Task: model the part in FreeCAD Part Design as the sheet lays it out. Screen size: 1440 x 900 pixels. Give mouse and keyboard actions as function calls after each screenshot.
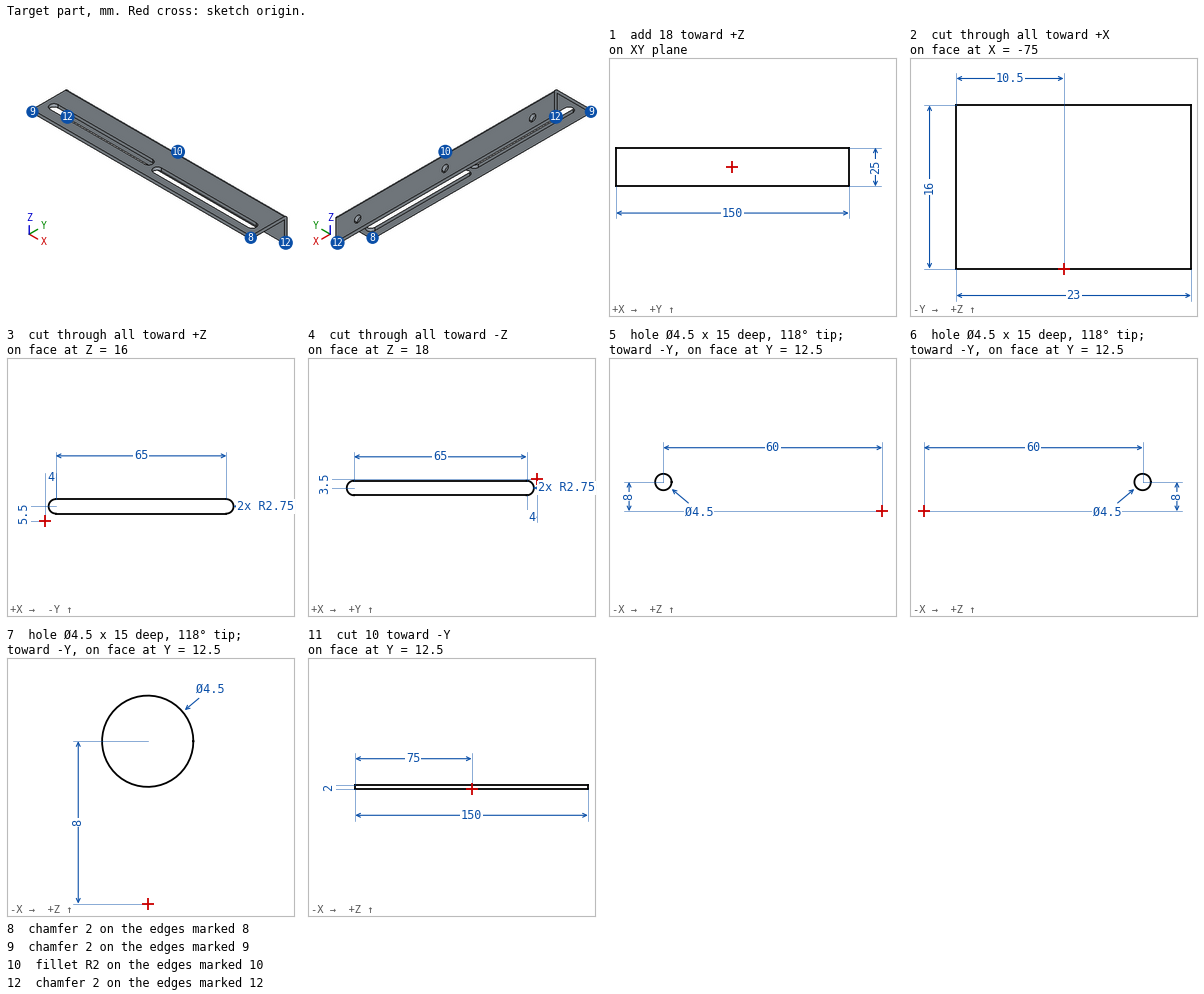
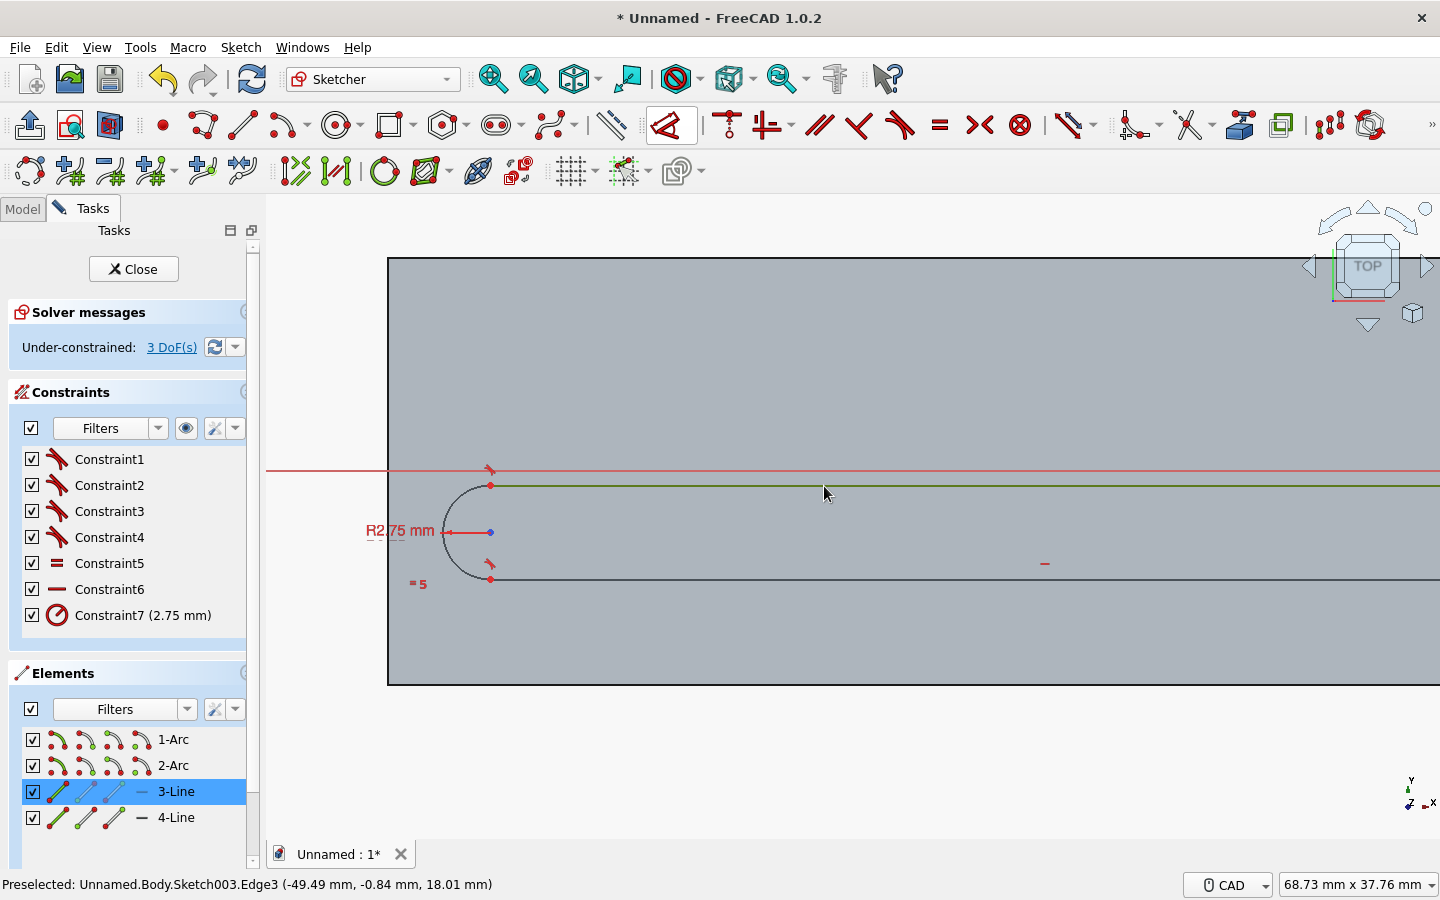
key(l)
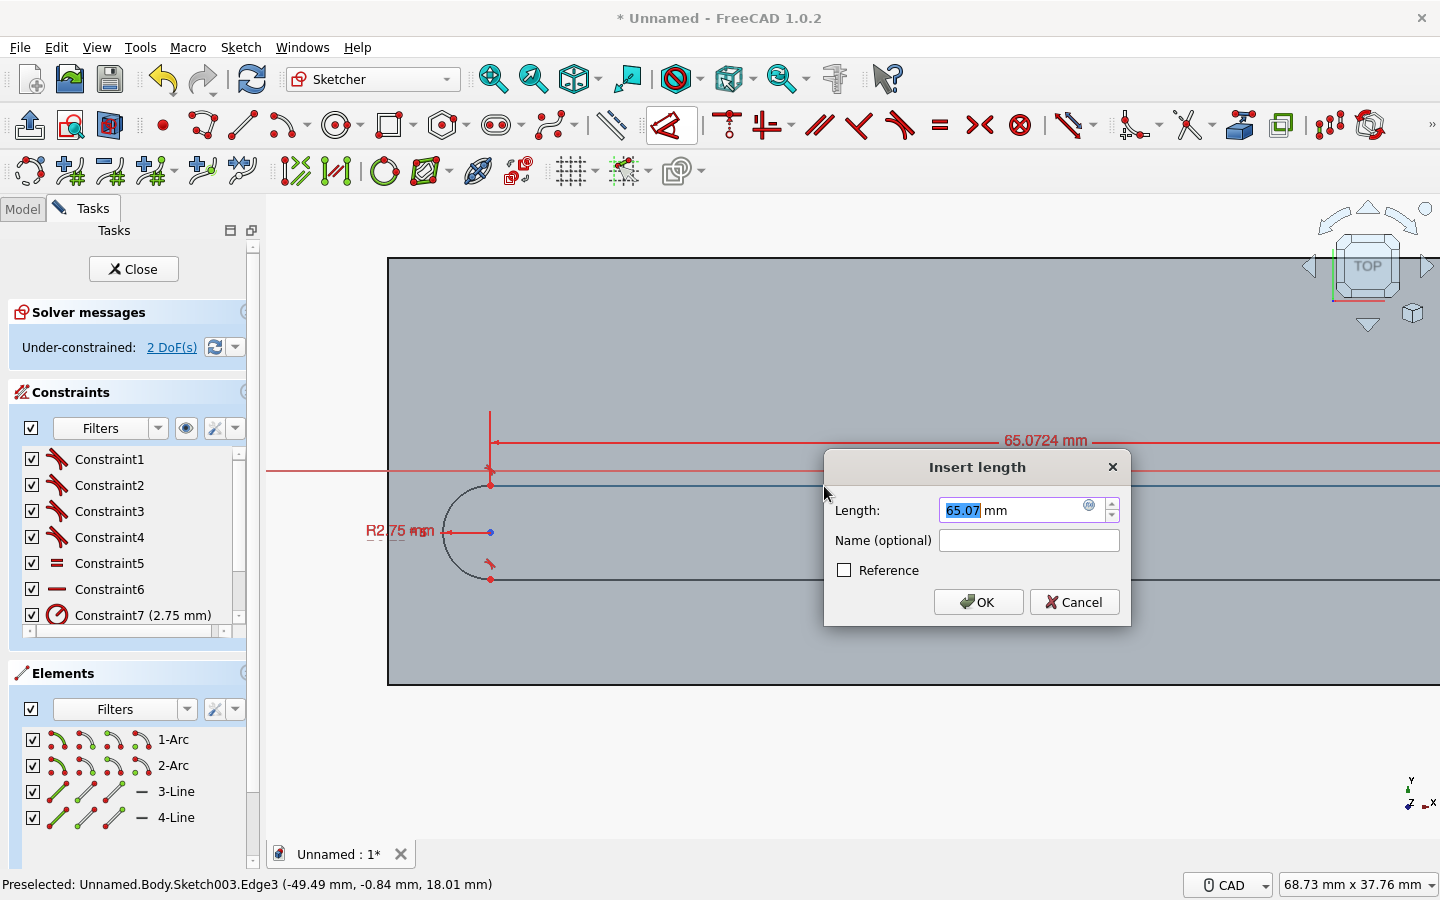
text(65)
key(Return)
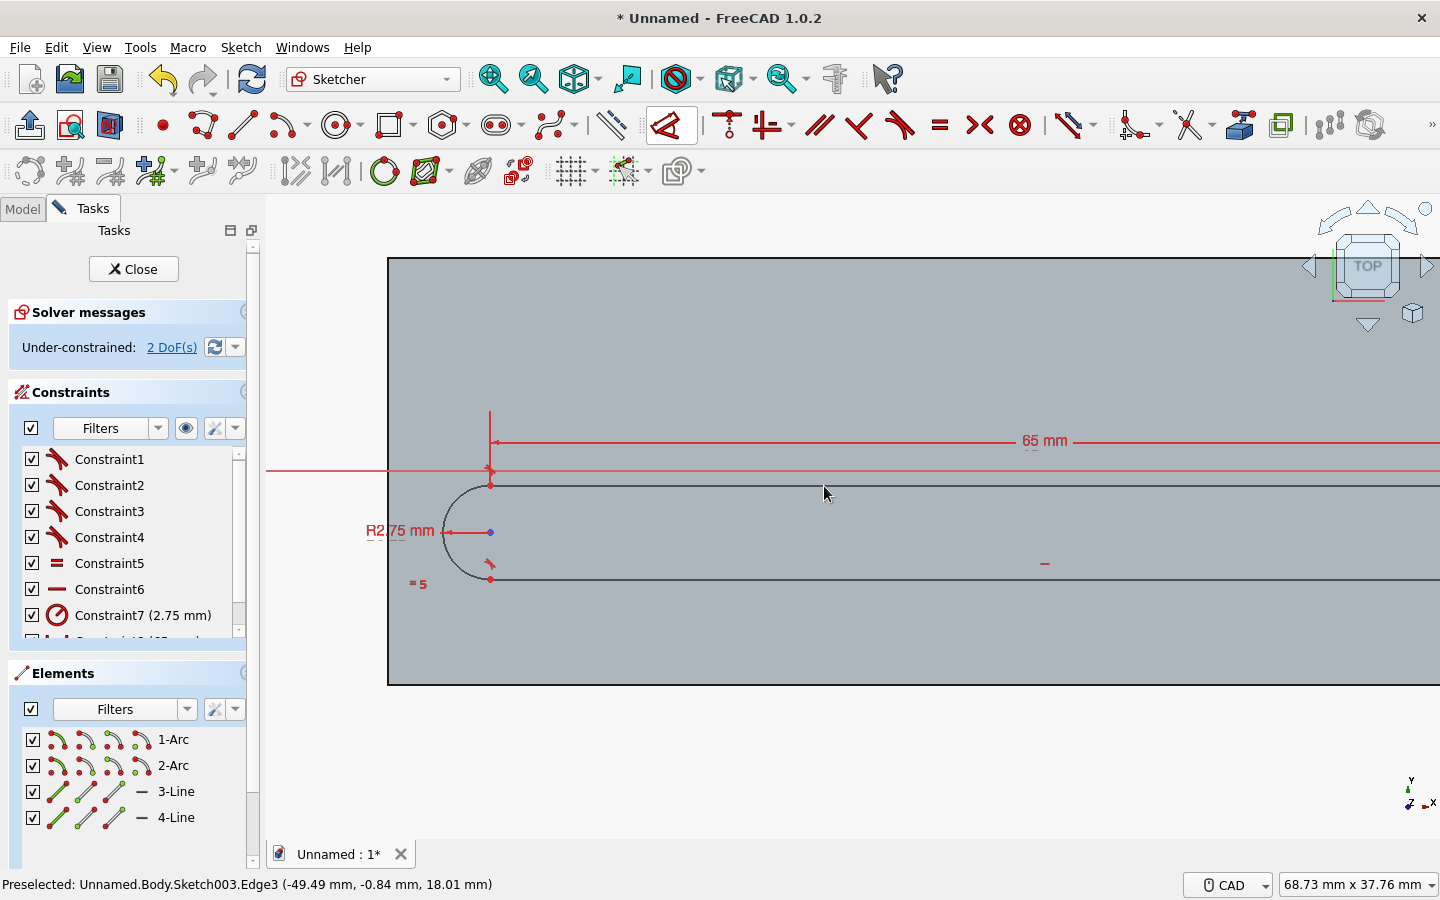
scroll(454, 507, down, 3)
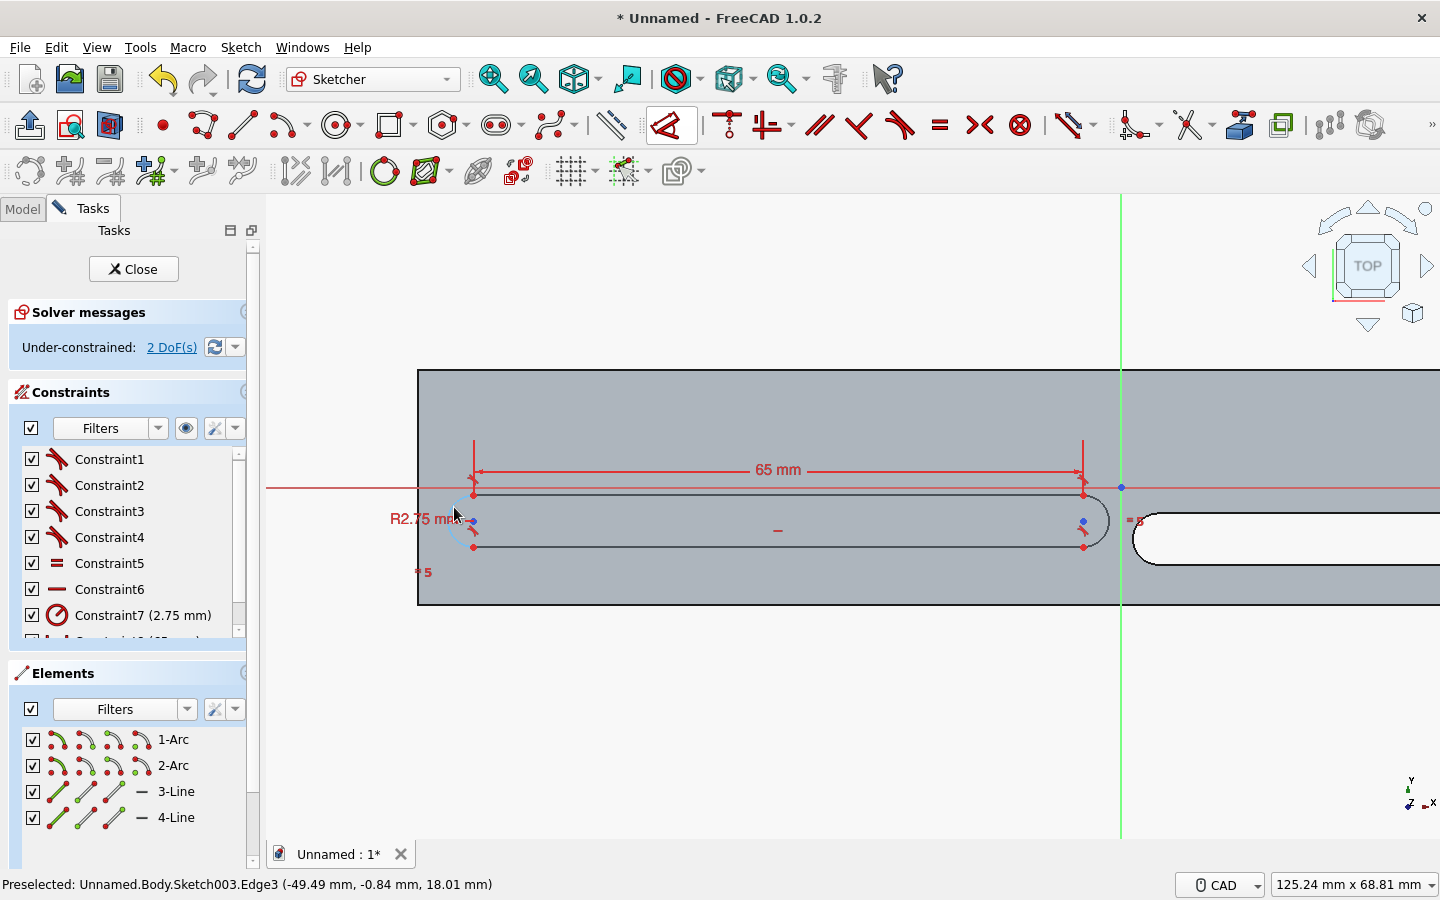
click(1083, 547)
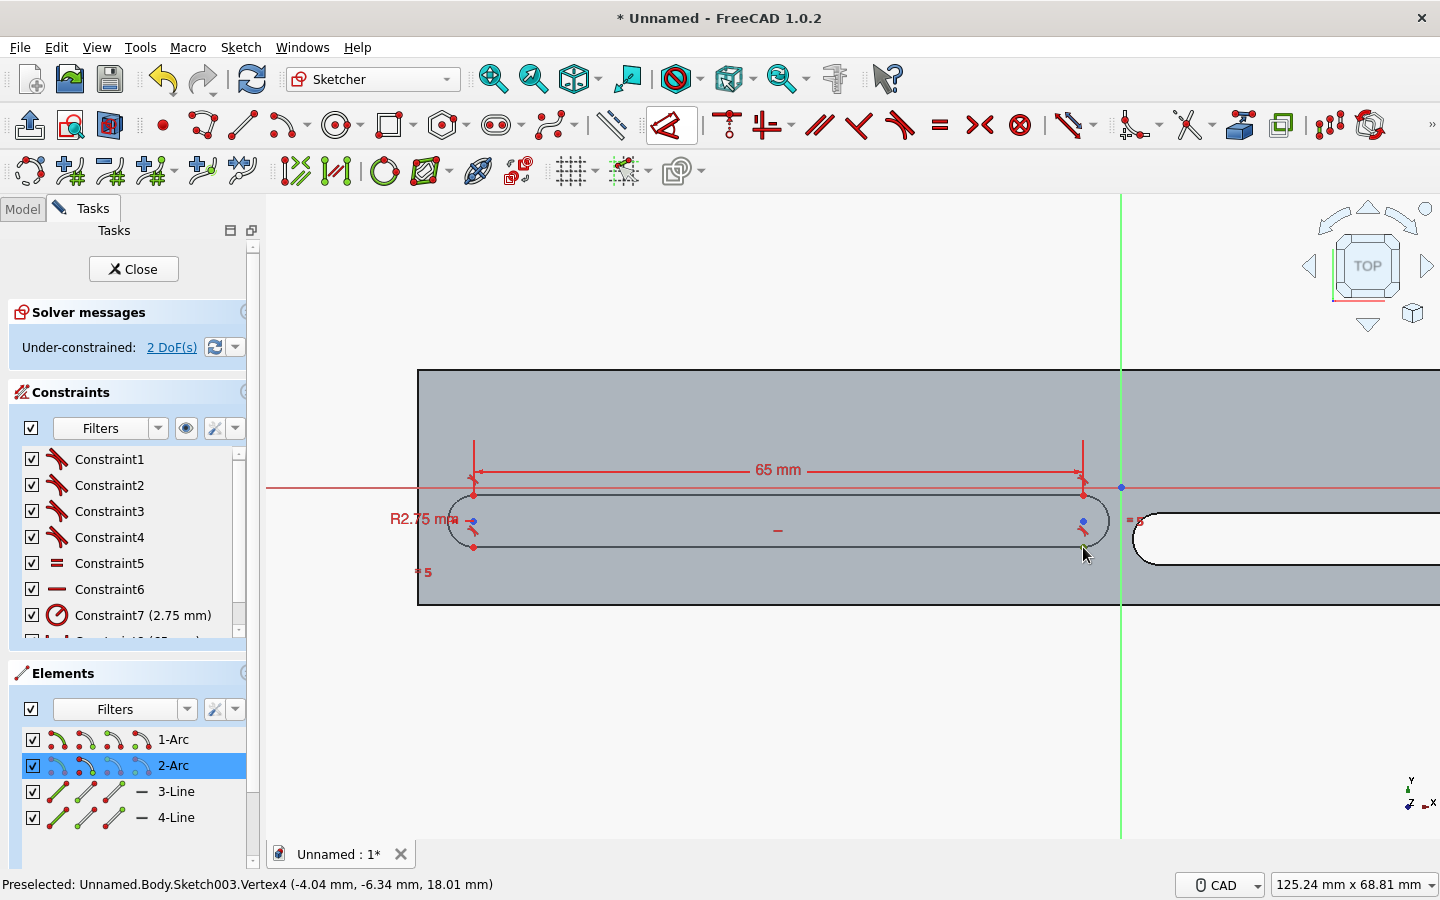
click(692, 126)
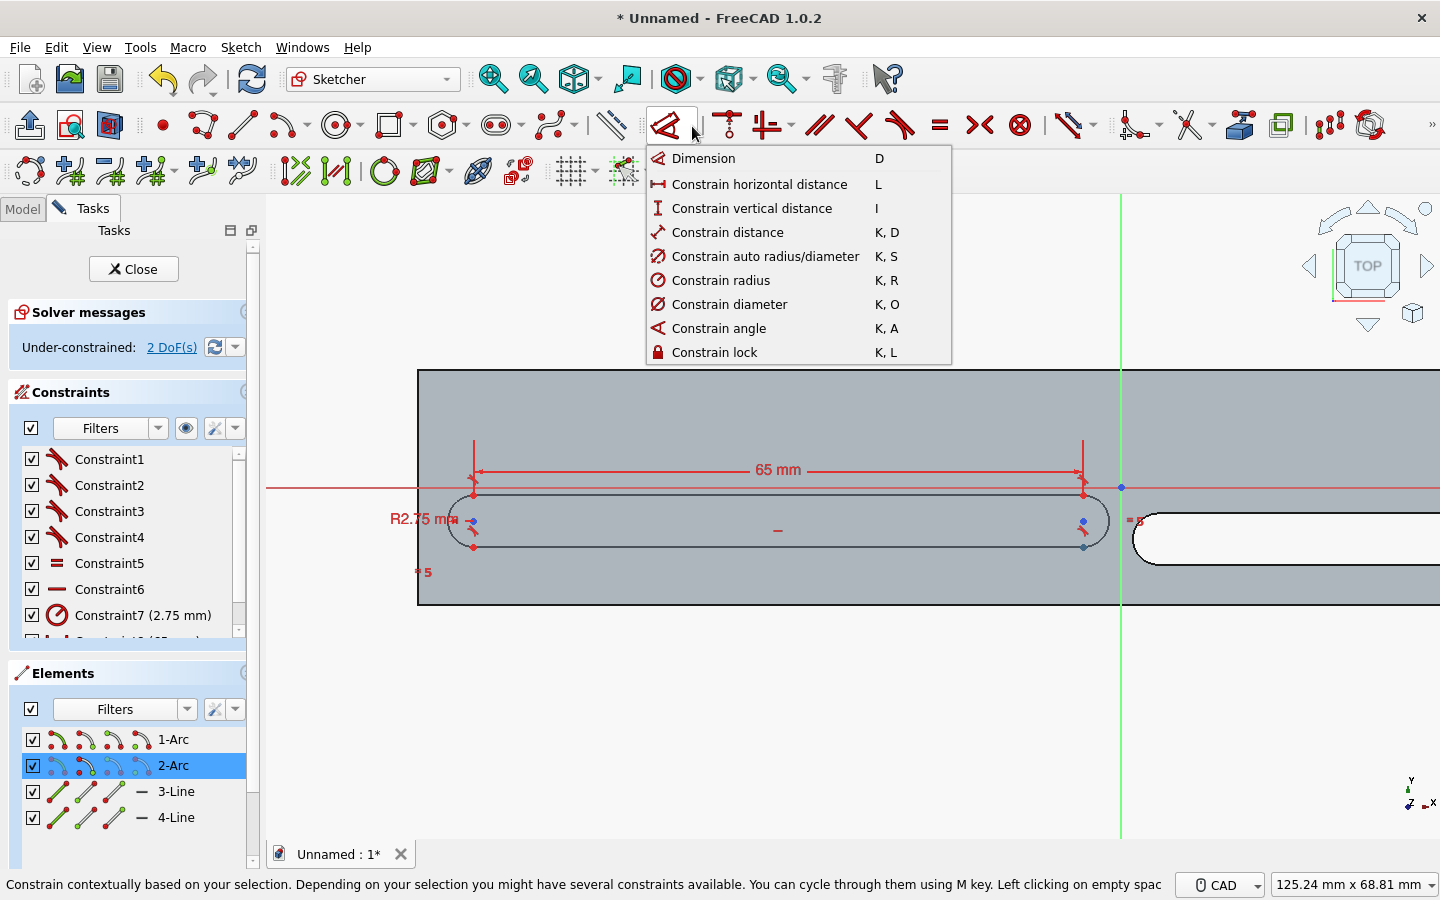
click(799, 184)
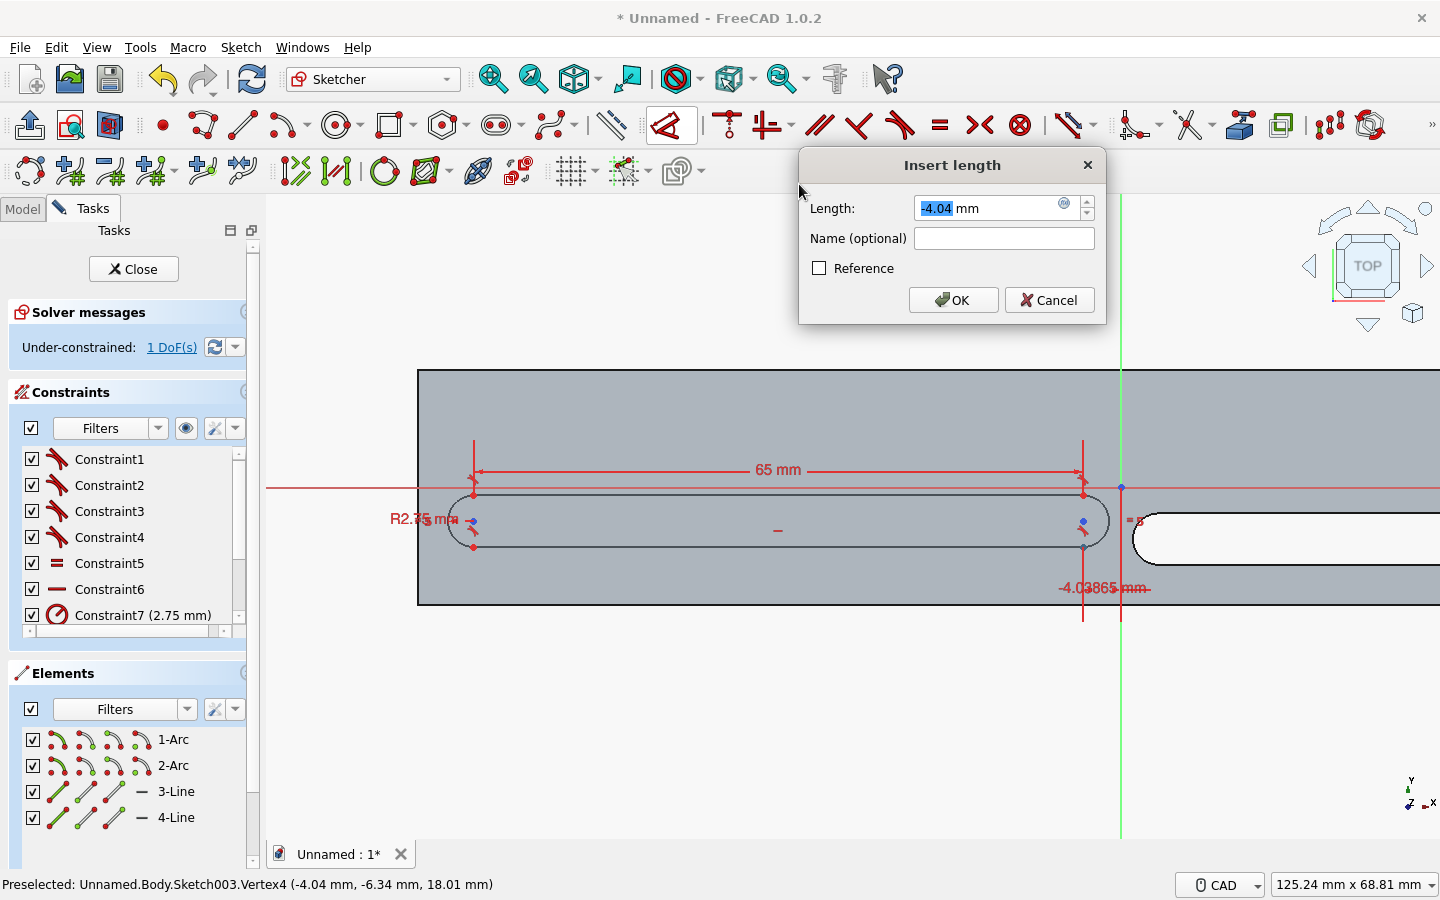
text(-4)
key(Return)